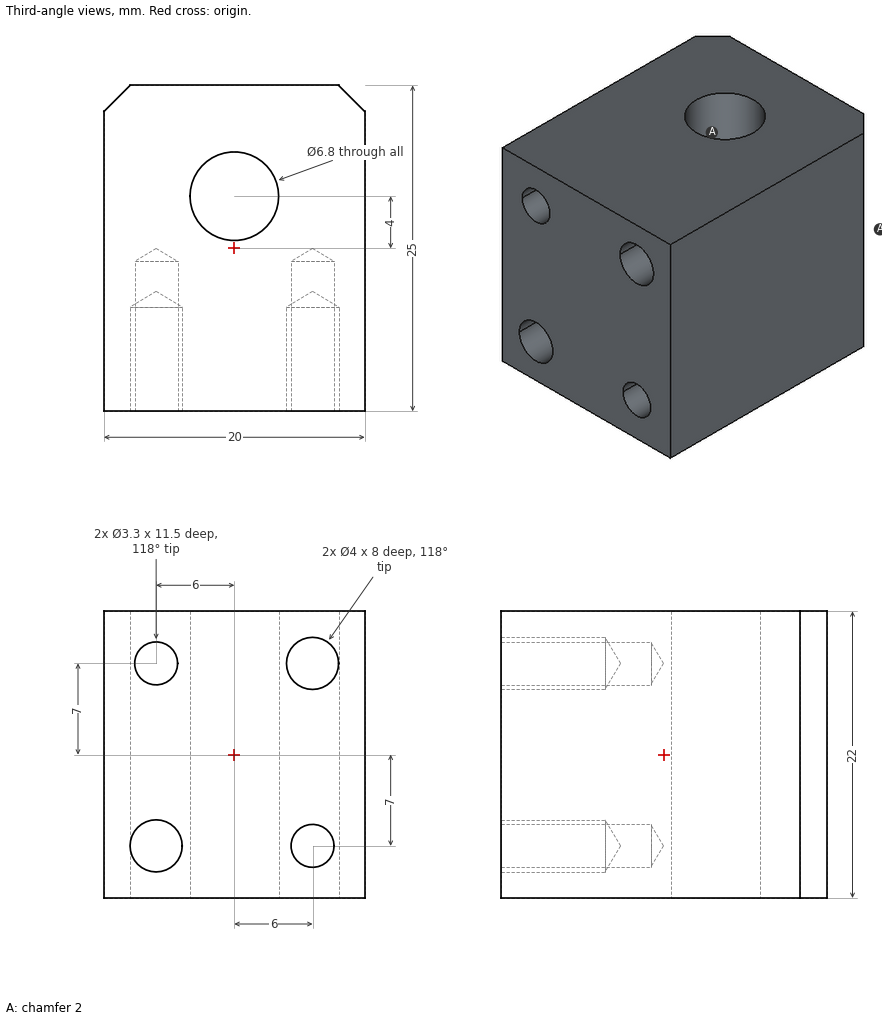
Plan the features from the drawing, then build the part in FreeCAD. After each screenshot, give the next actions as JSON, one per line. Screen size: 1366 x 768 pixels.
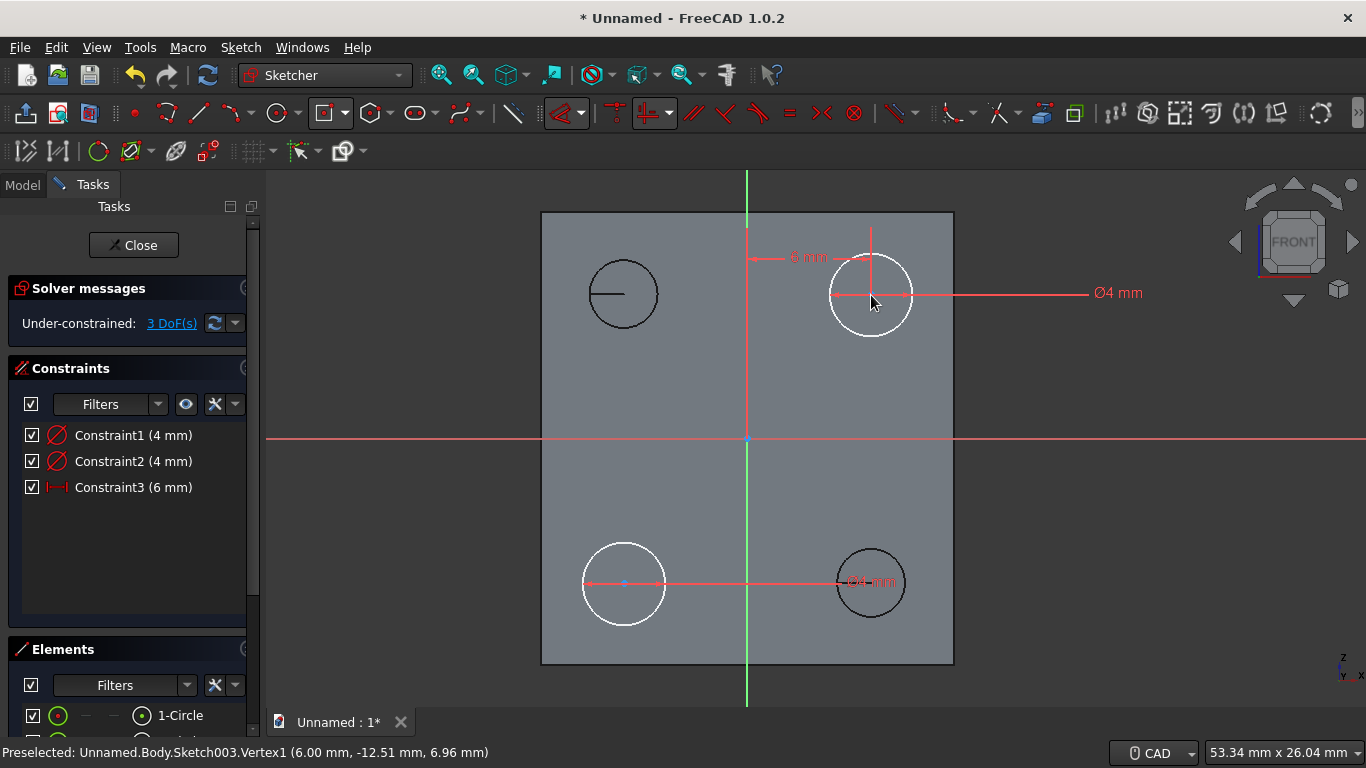
{"action": "left_click", "coordinate": [871, 295]}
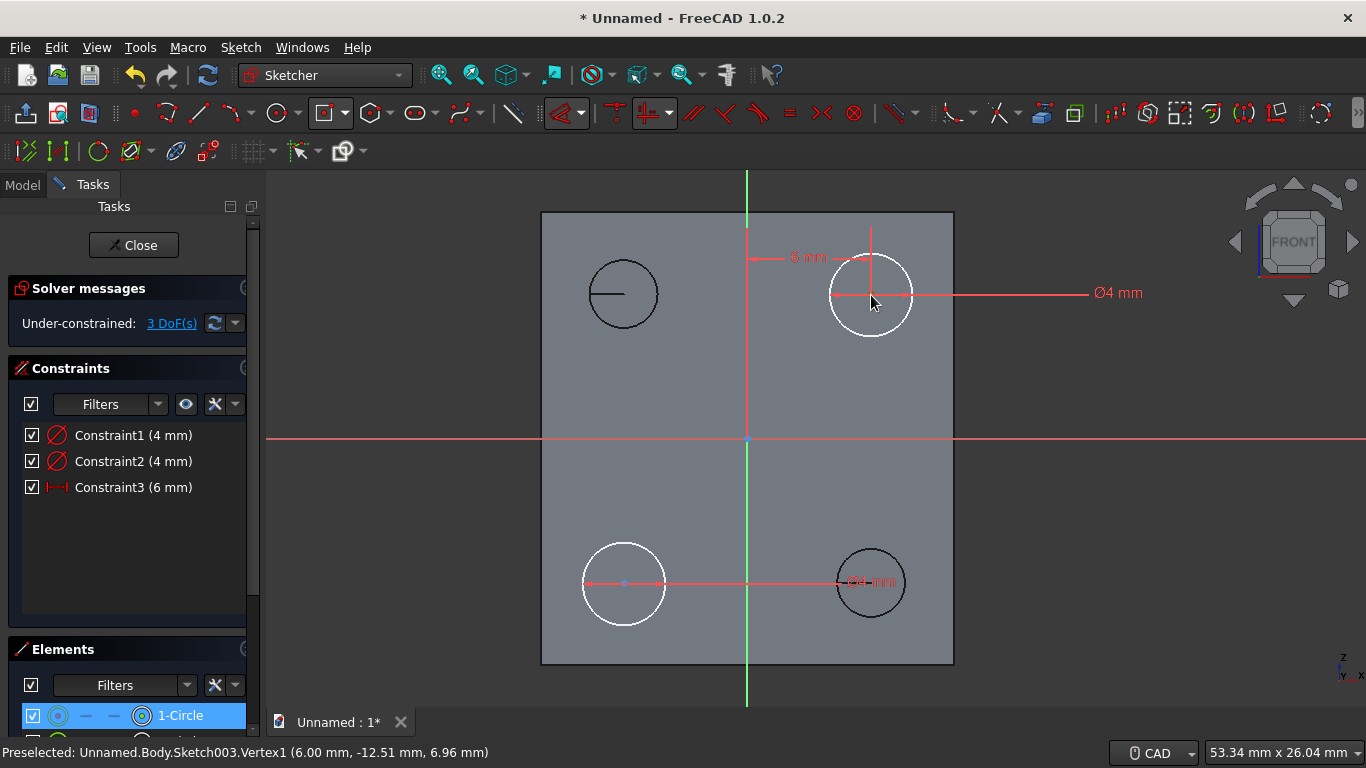
{"action": "key", "text": "i"}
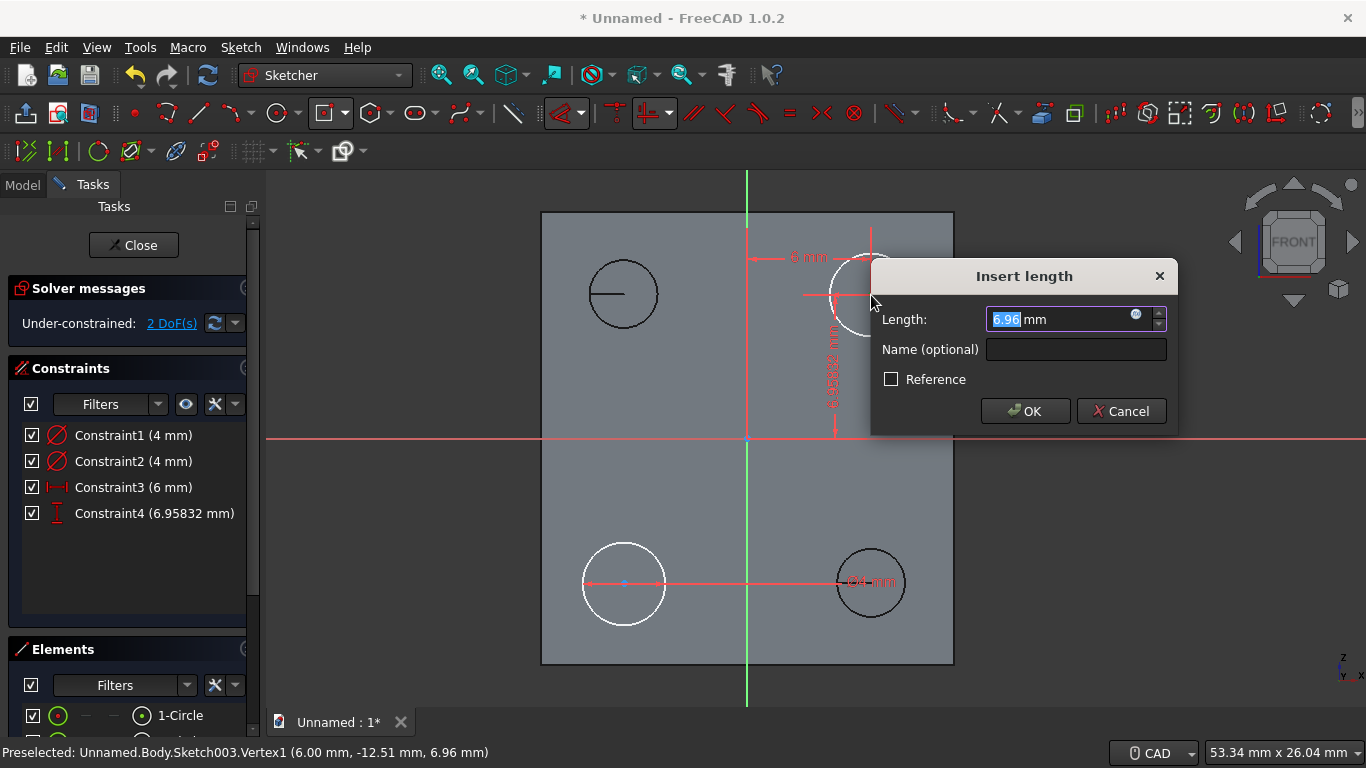
{"action": "type", "text": "7"}
{"action": "key", "text": "Return"}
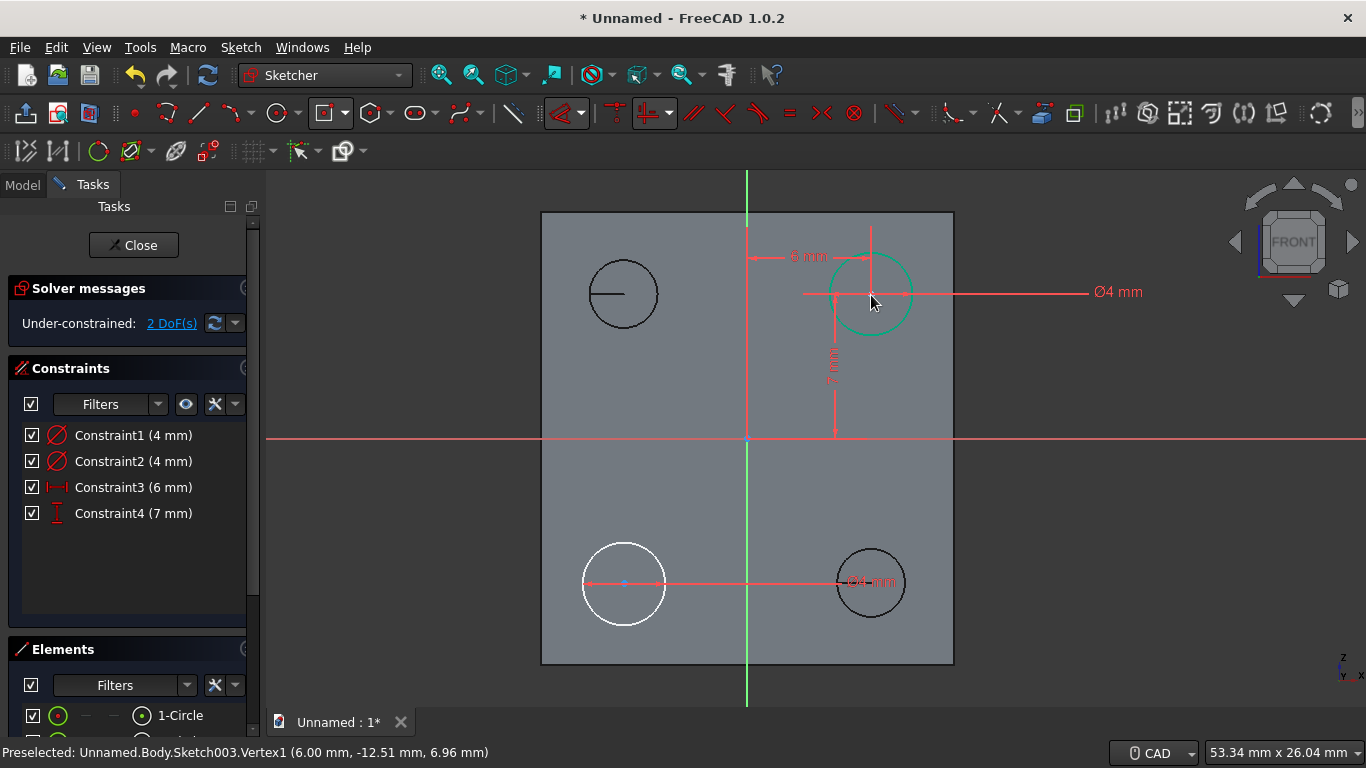
{"action": "left_click", "coordinate": [624, 584]}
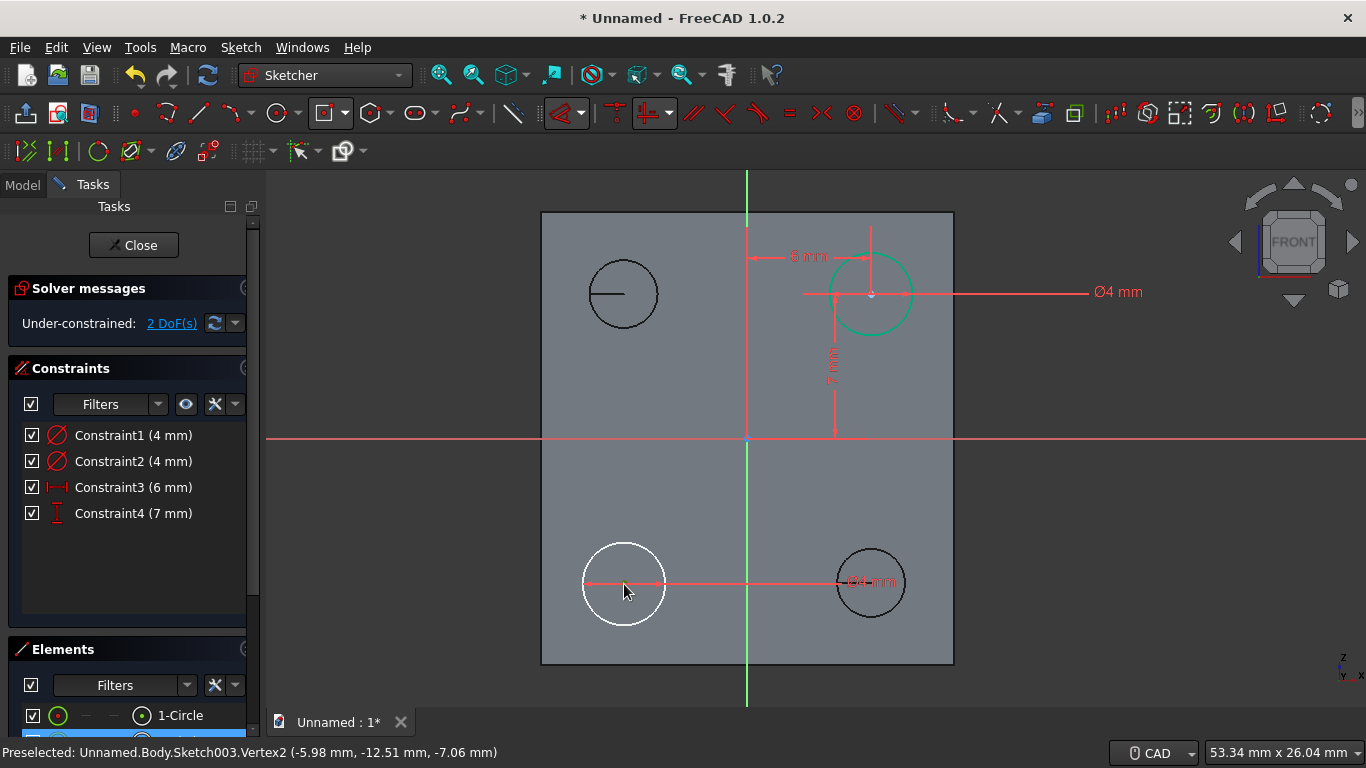
{"action": "key", "text": "l"}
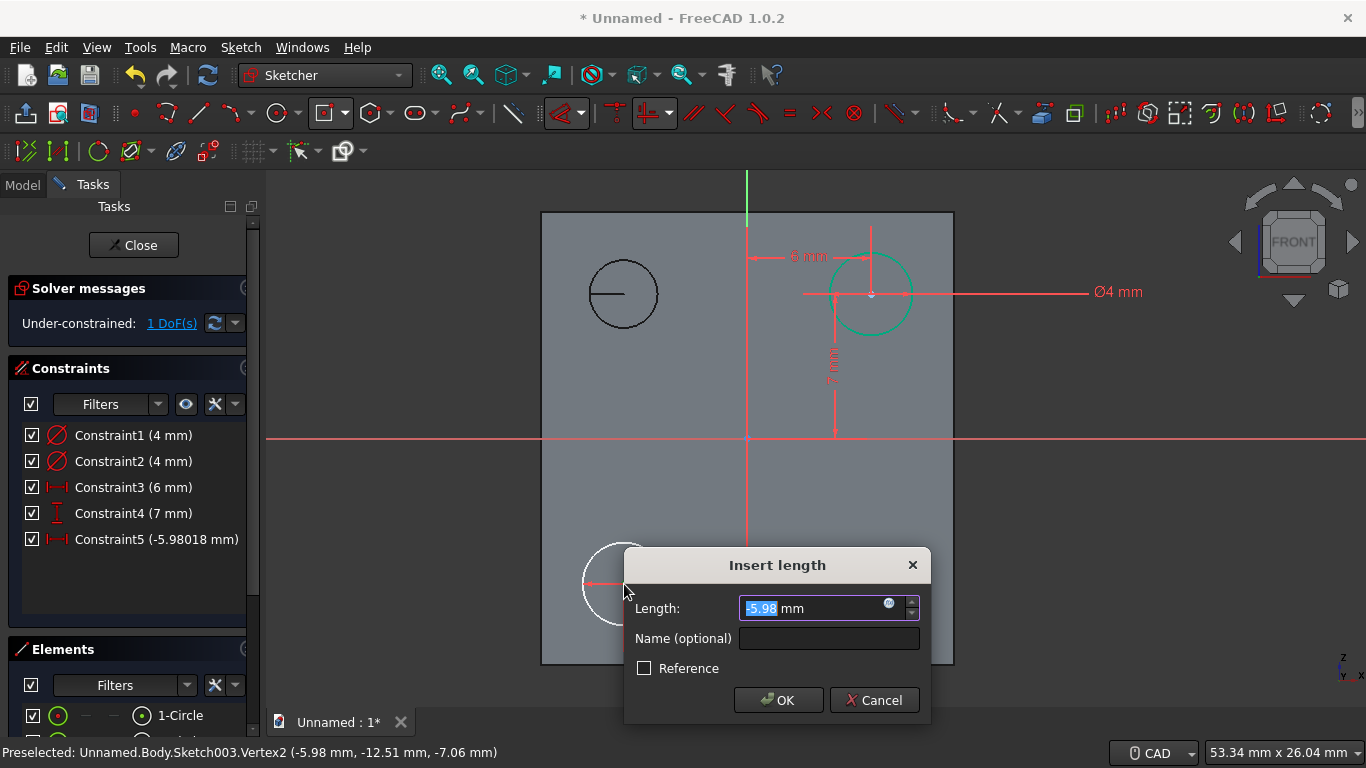
{"action": "type", "text": "-6"}
{"action": "key", "text": "Return"}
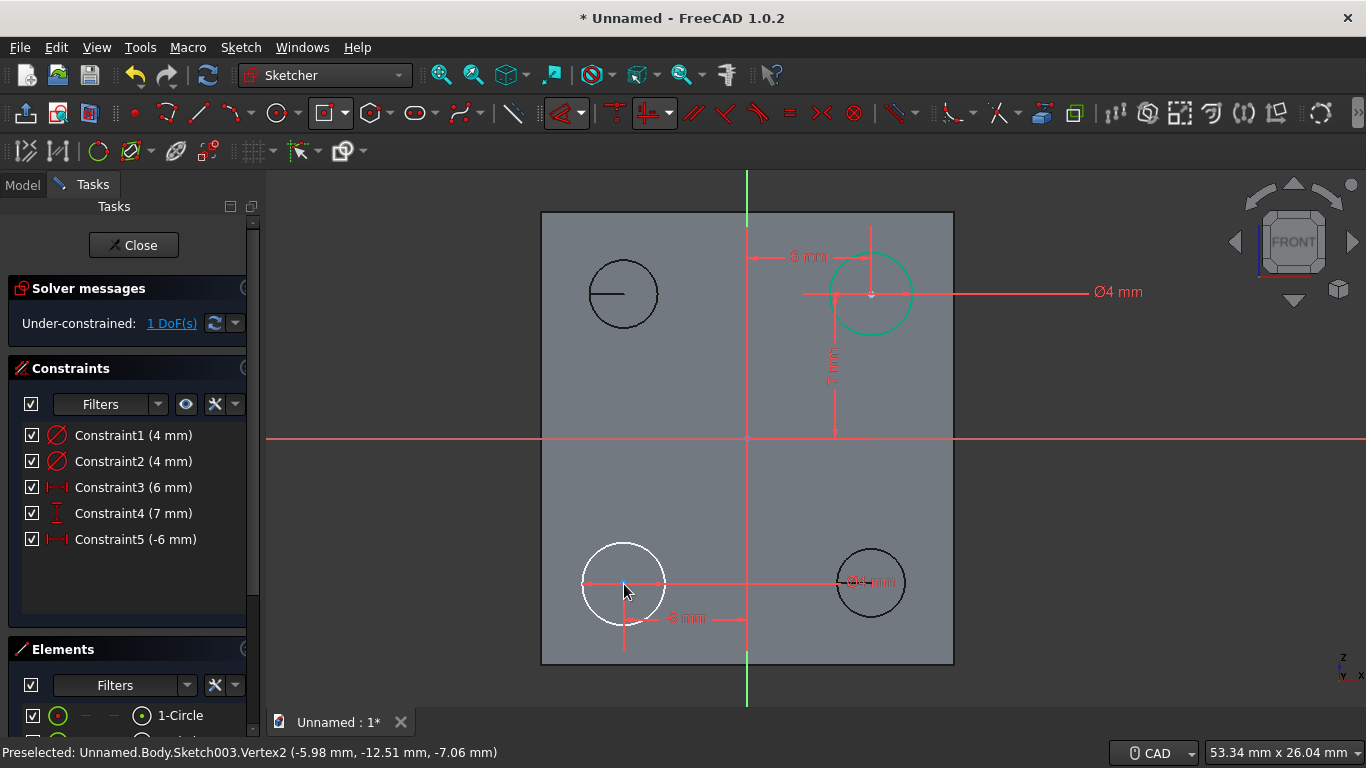
{"action": "left_click", "coordinate": [624, 584]}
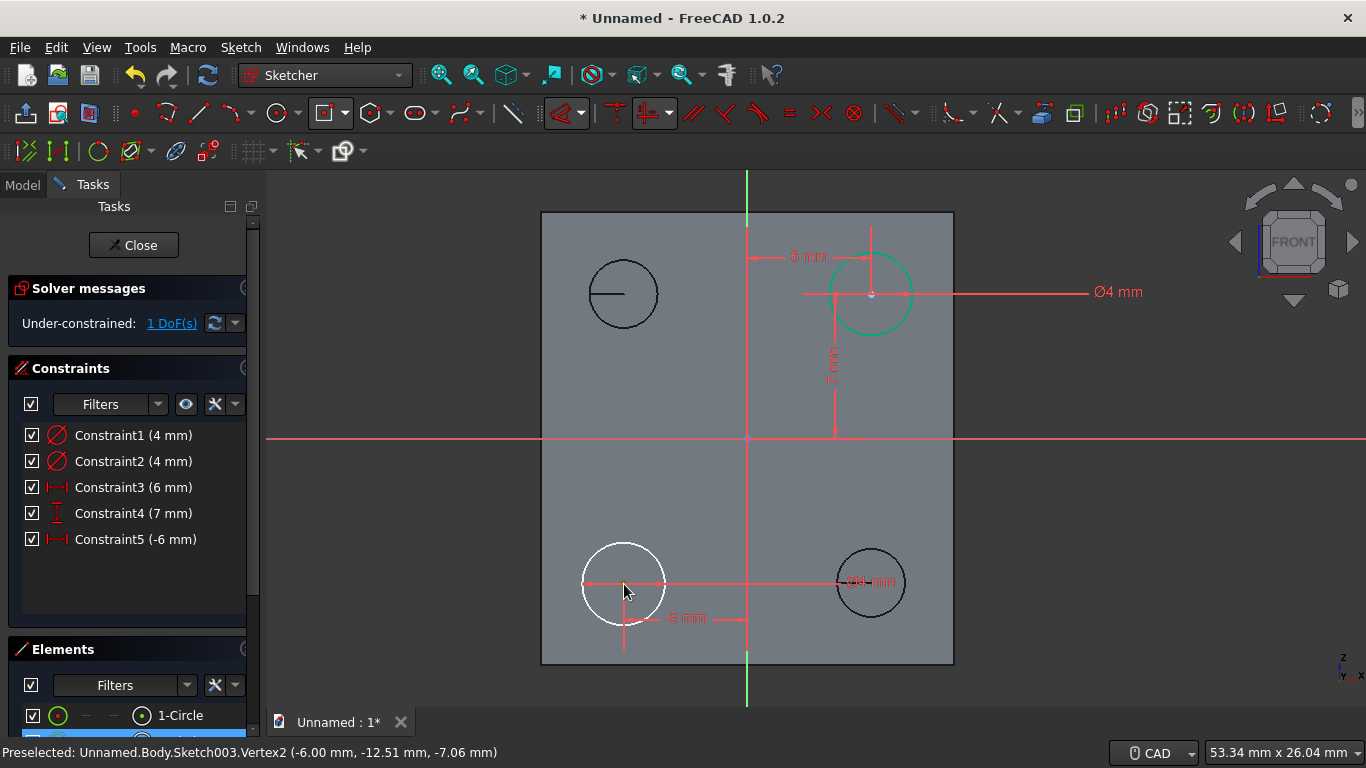
{"action": "left_click", "coordinate": [584, 114]}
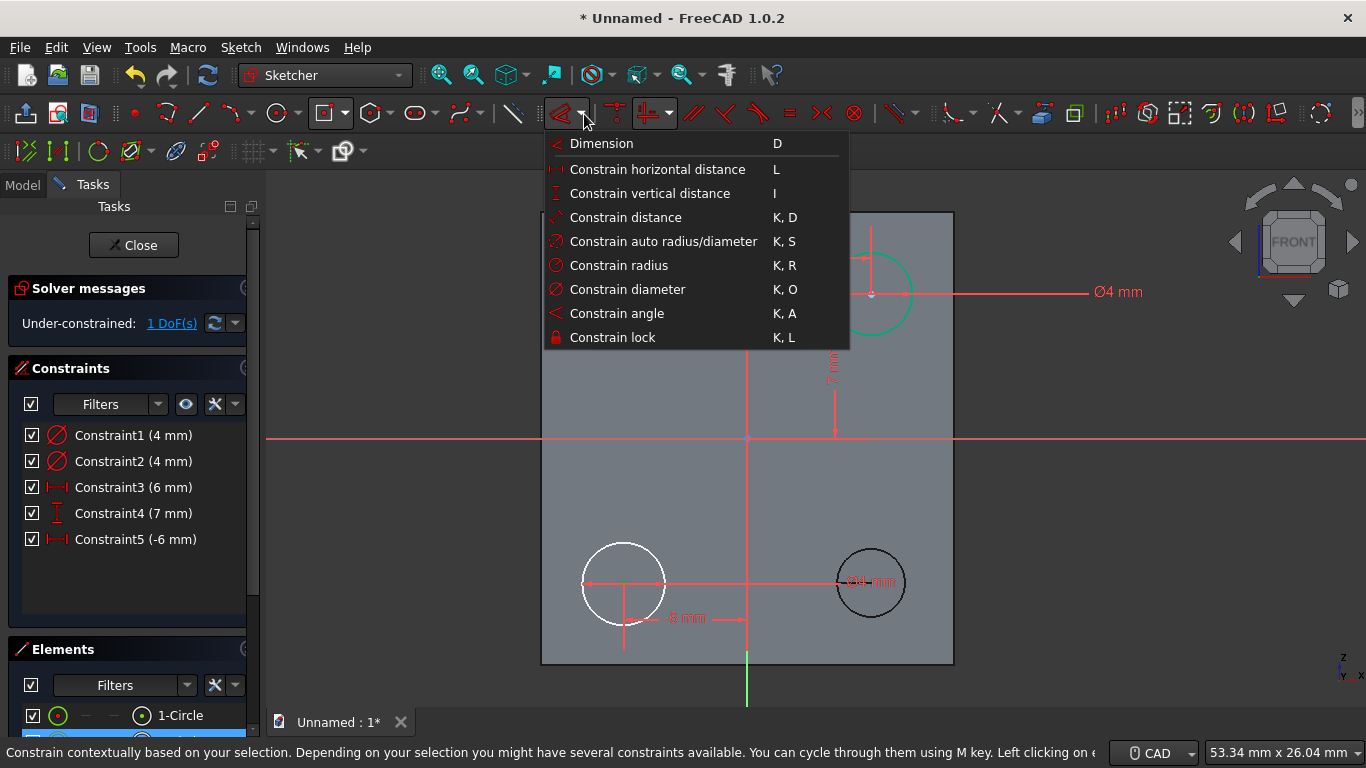
{"action": "left_click", "coordinate": [697, 193]}